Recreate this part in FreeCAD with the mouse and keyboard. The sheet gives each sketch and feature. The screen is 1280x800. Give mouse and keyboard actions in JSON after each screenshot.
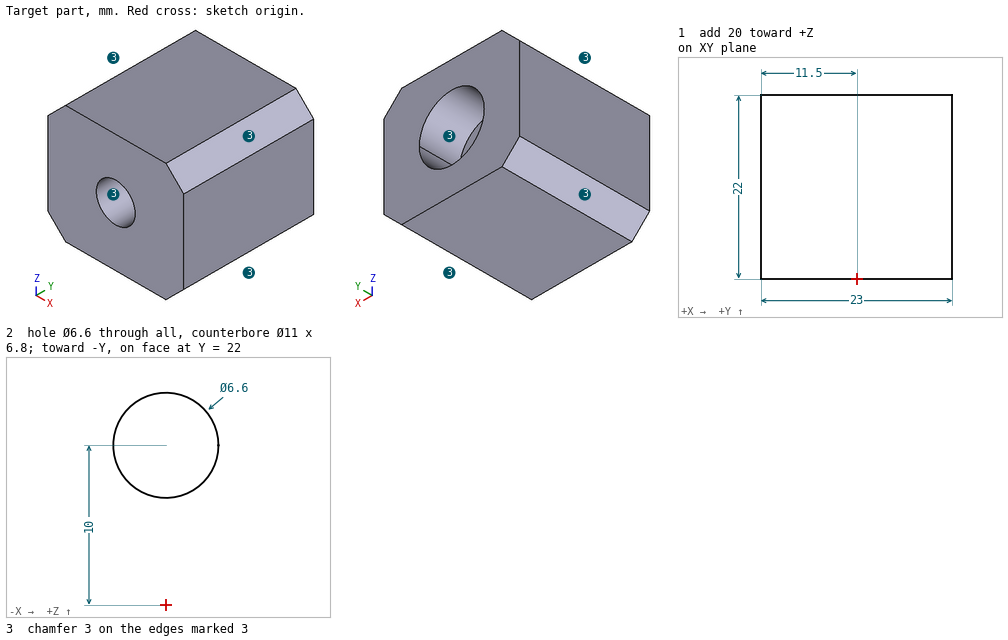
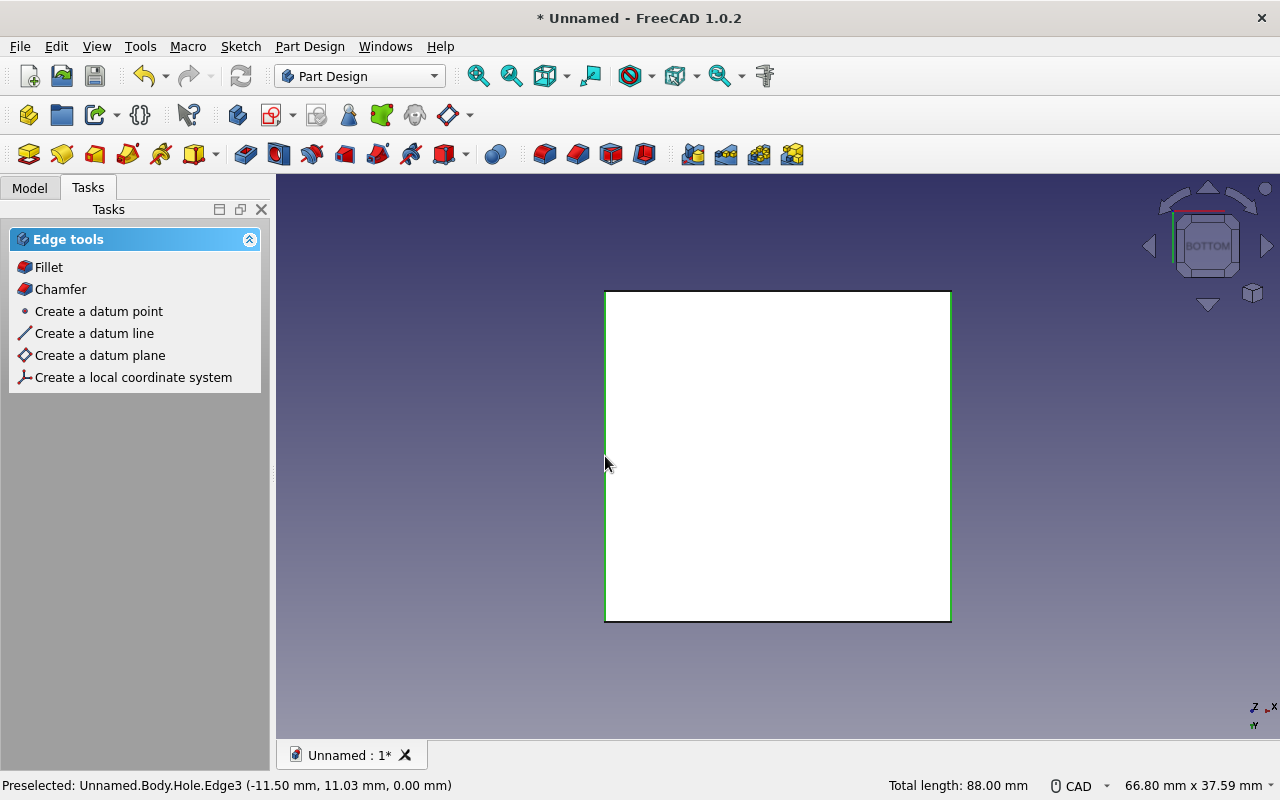
{"action": "left_click", "coordinate": [578, 154]}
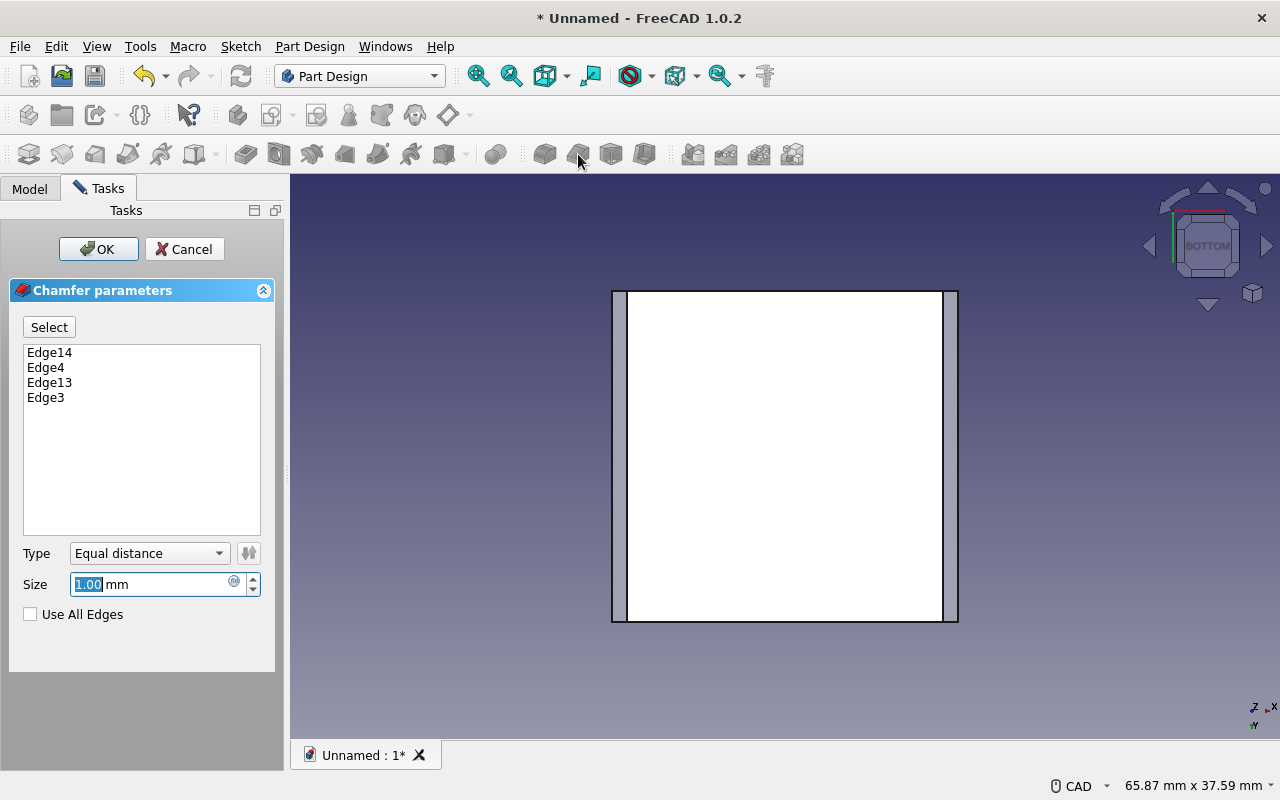
{"action": "type", "text": "3"}
{"action": "key", "text": "Tab"}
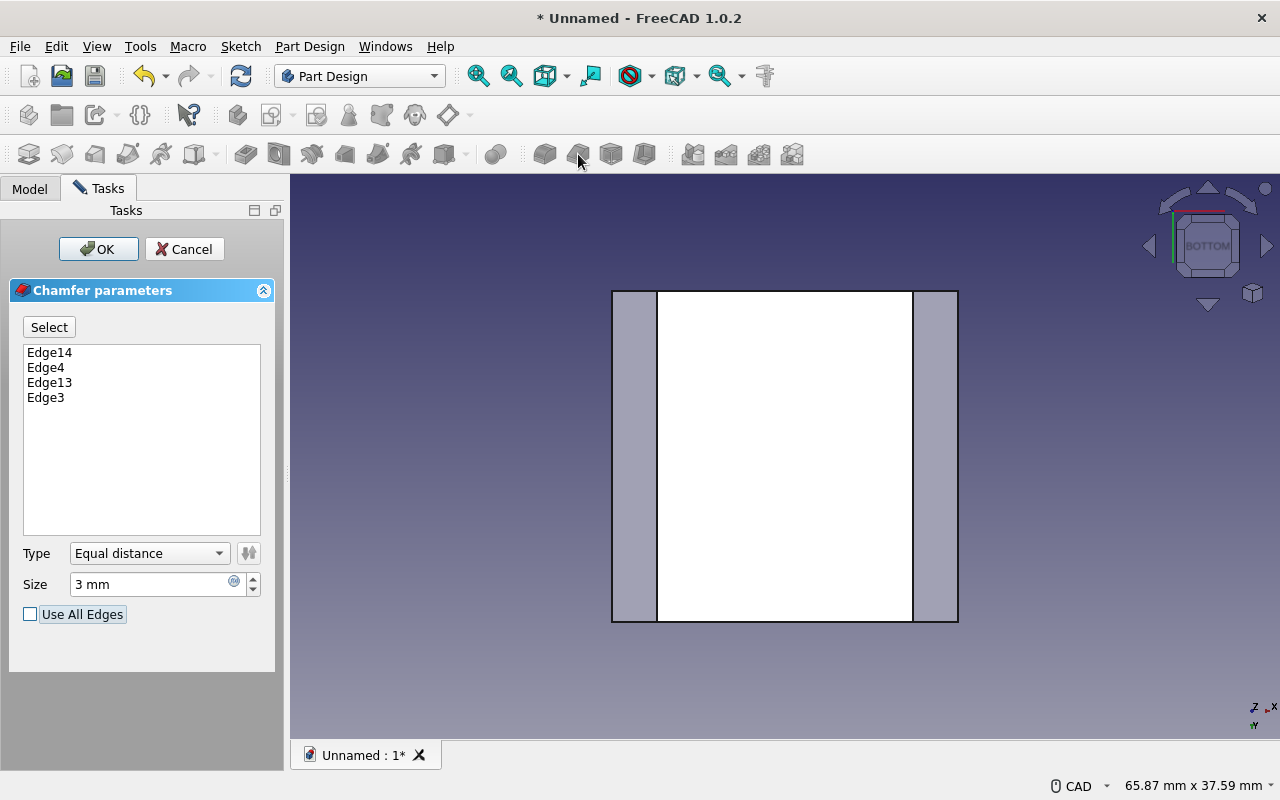
{"action": "left_click", "coordinate": [99, 249]}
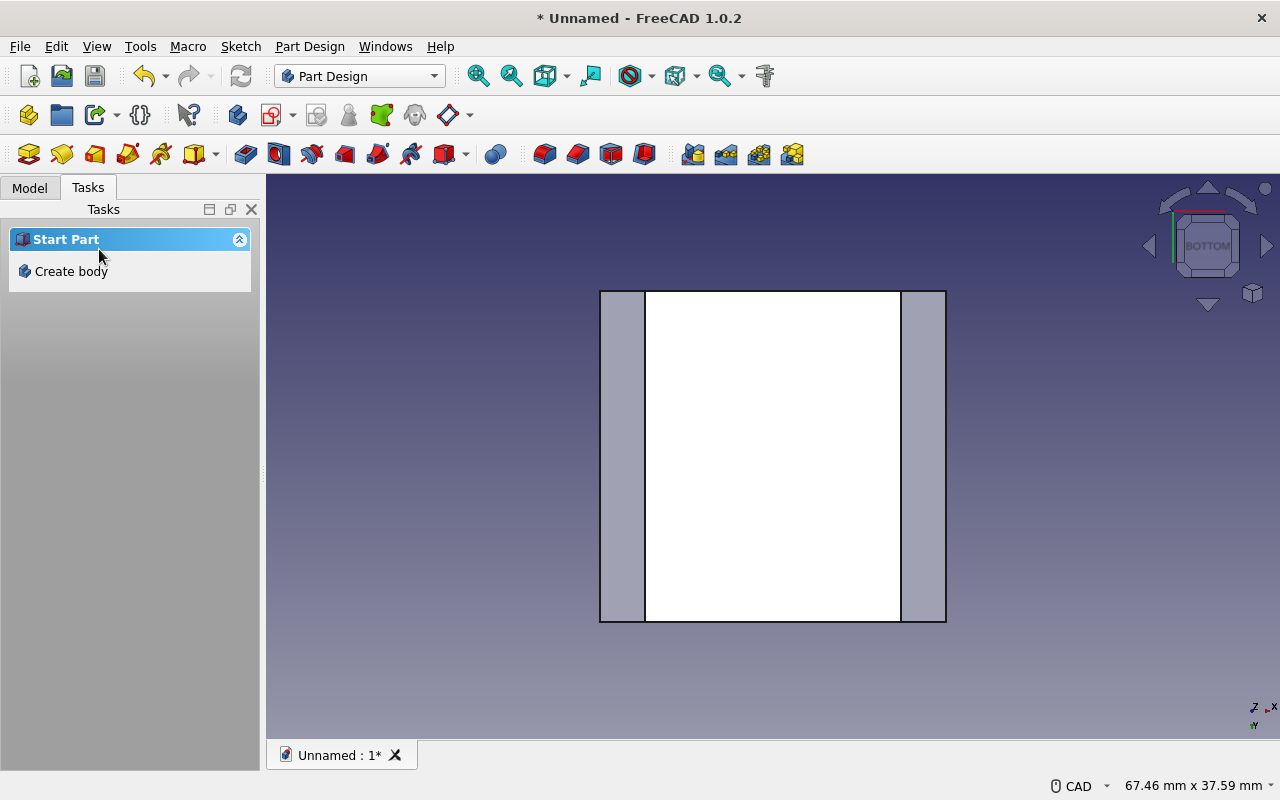
{"action": "key", "text": "0"}